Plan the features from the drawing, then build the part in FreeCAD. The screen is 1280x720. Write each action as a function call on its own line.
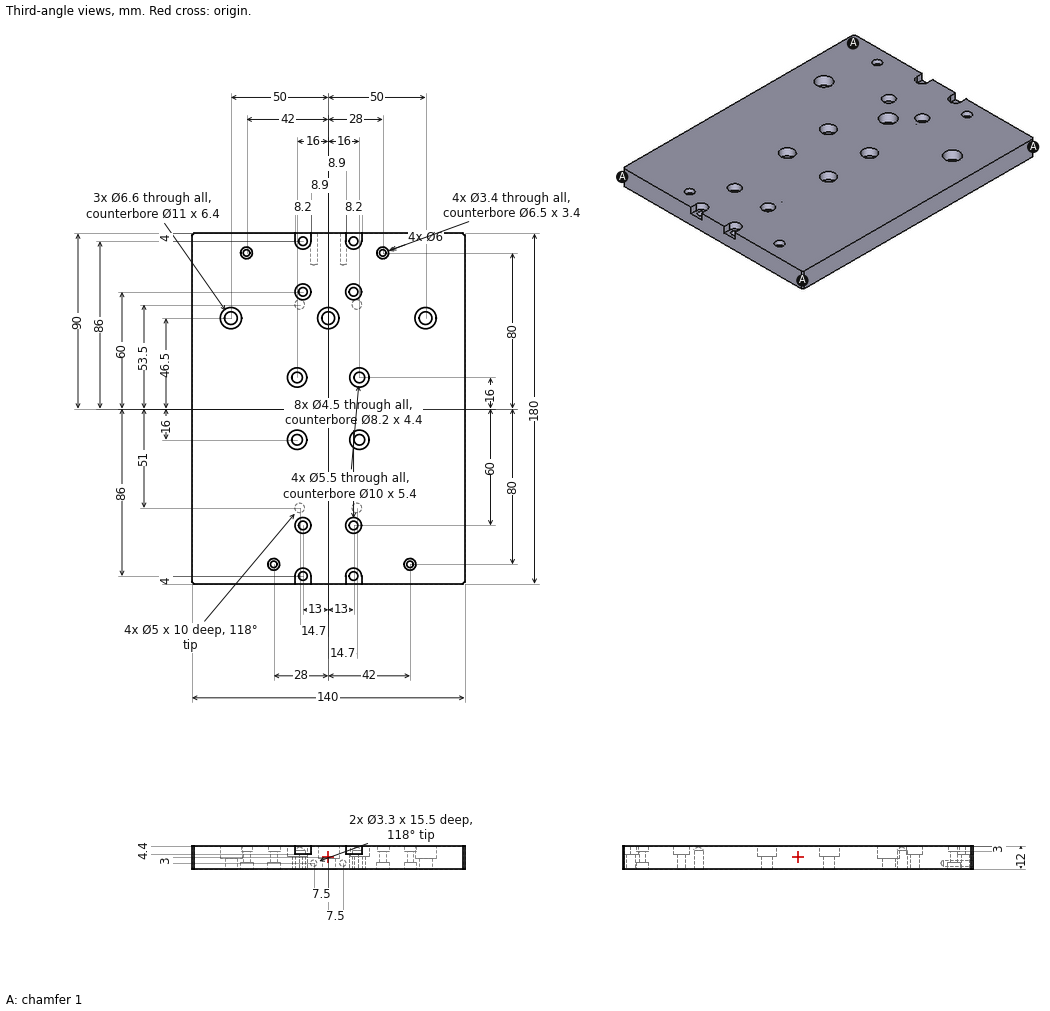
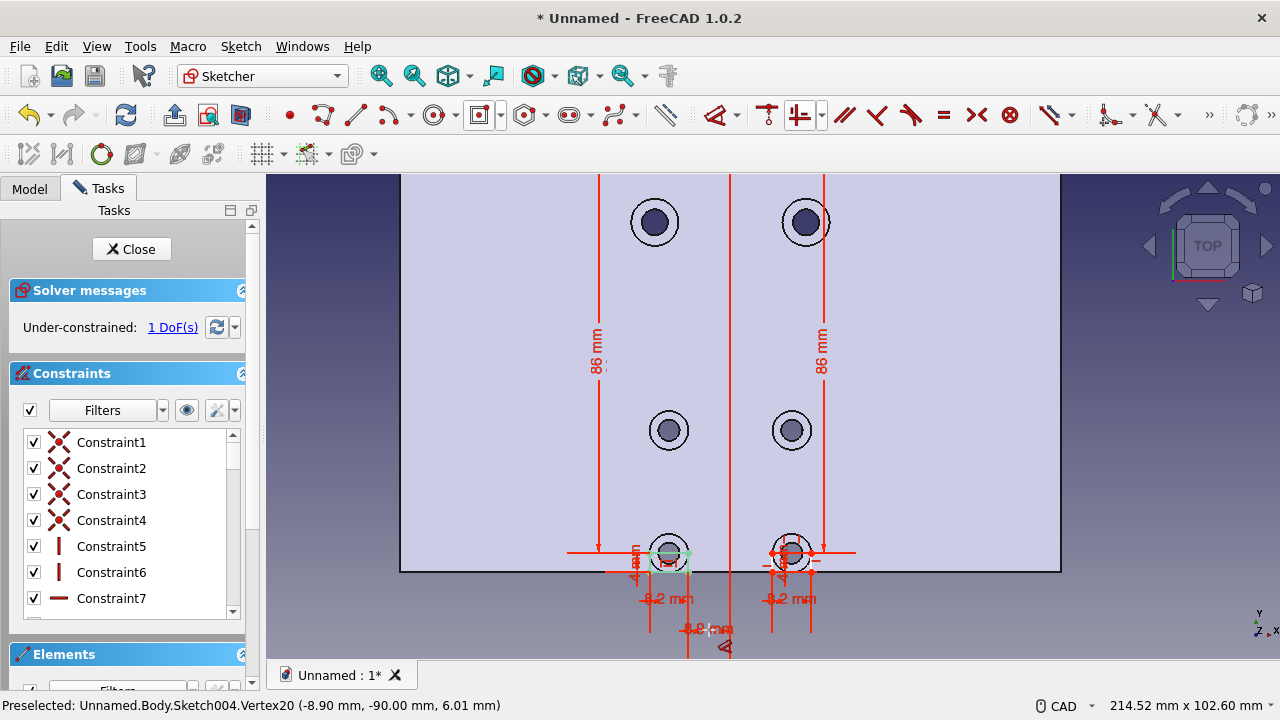
click(772, 553)
click(751, 587)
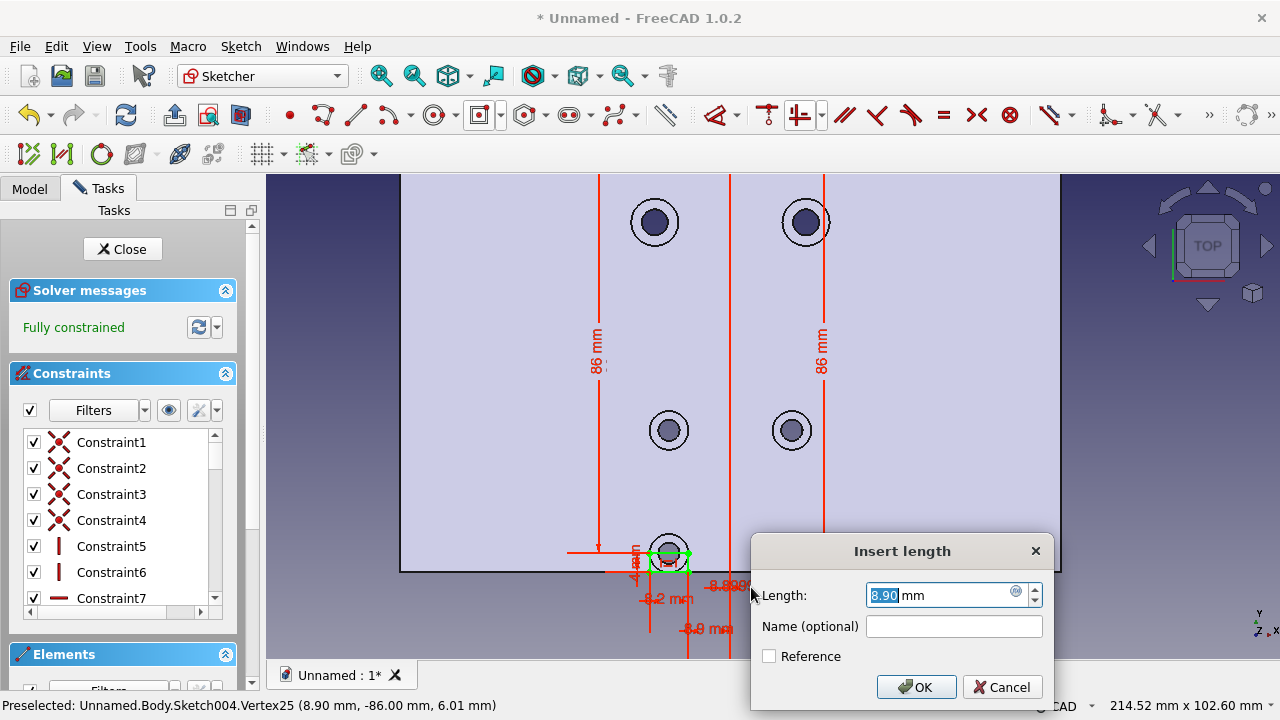
text(8.9)
key(Return)
key(Escape)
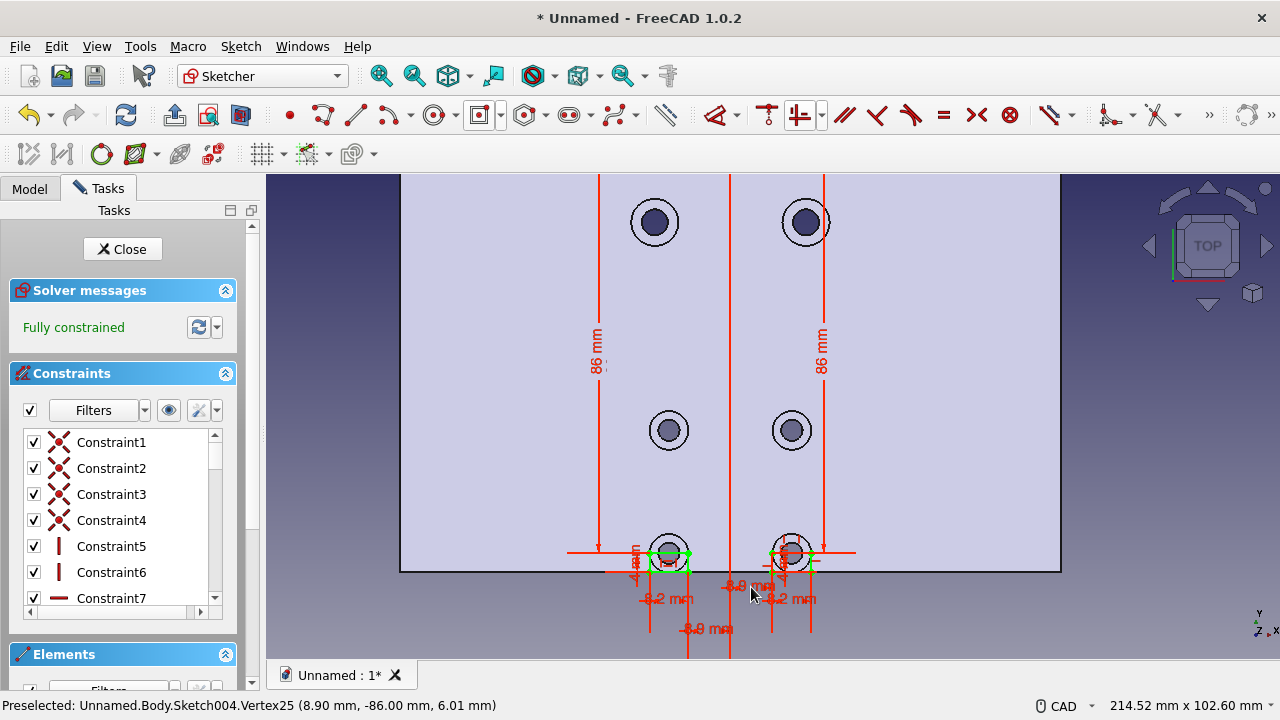
click(123, 249)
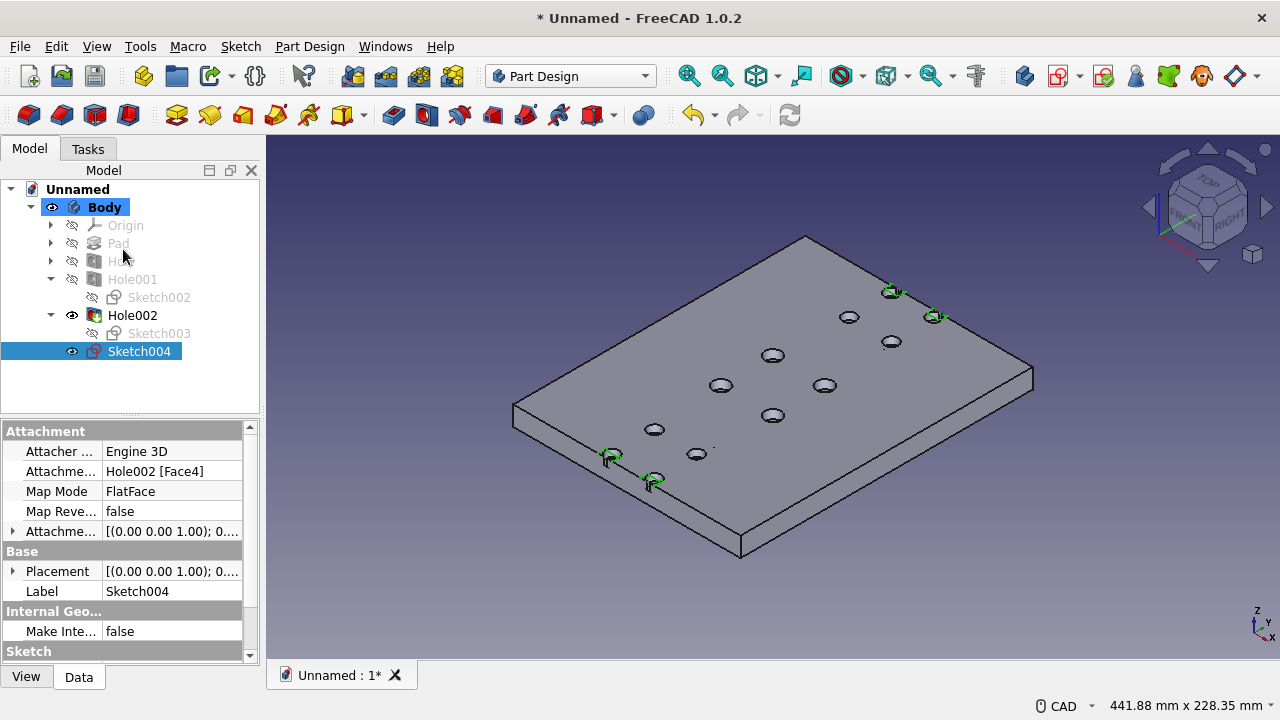
click(394, 116)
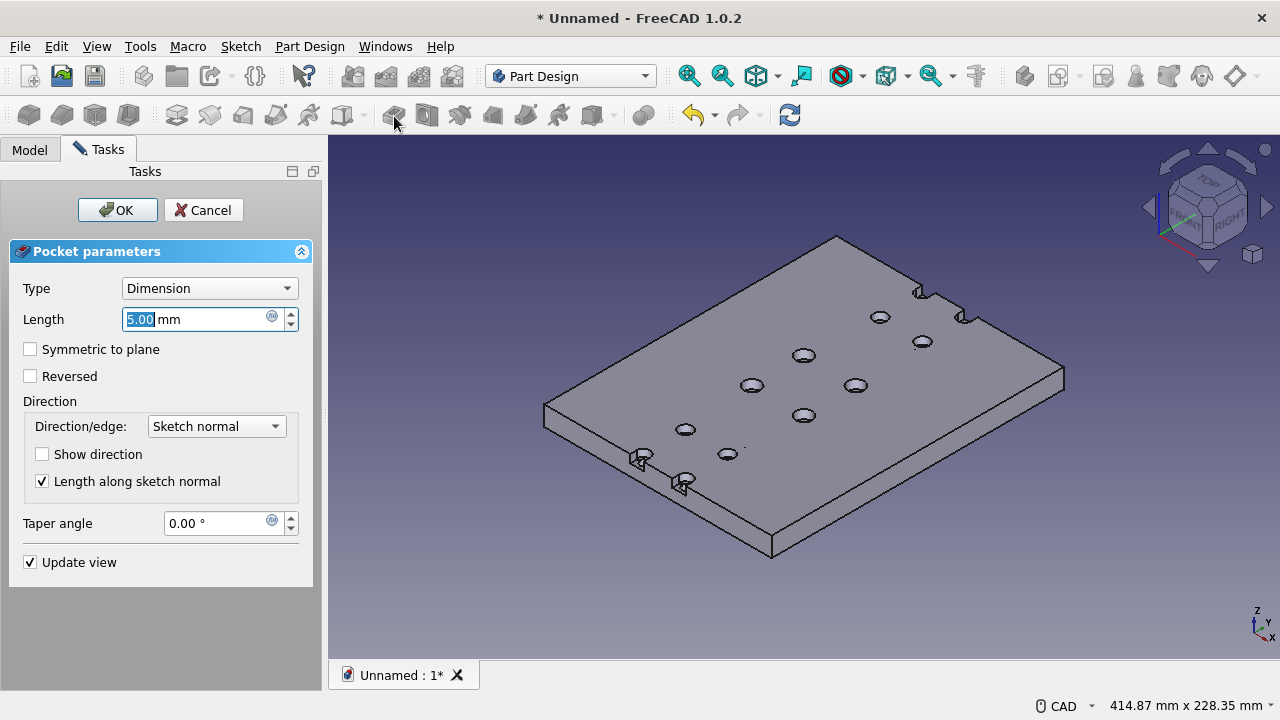
text(4.4)
key(Tab)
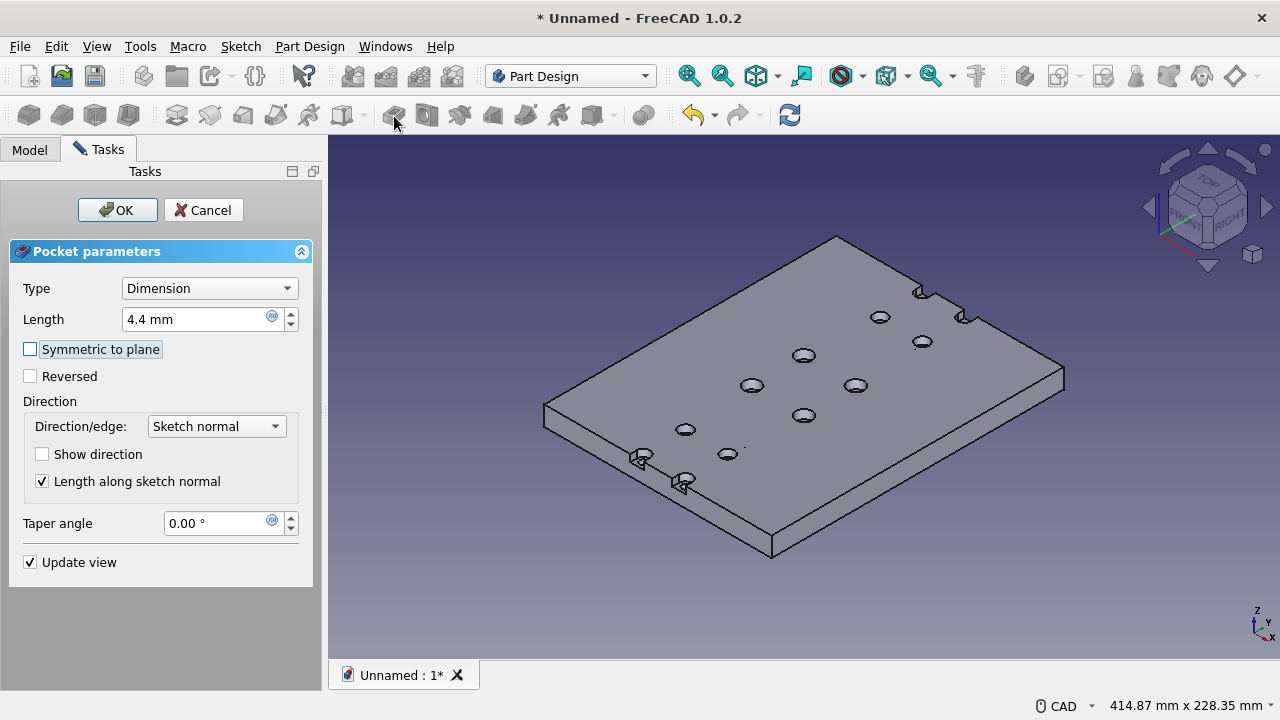
click(118, 210)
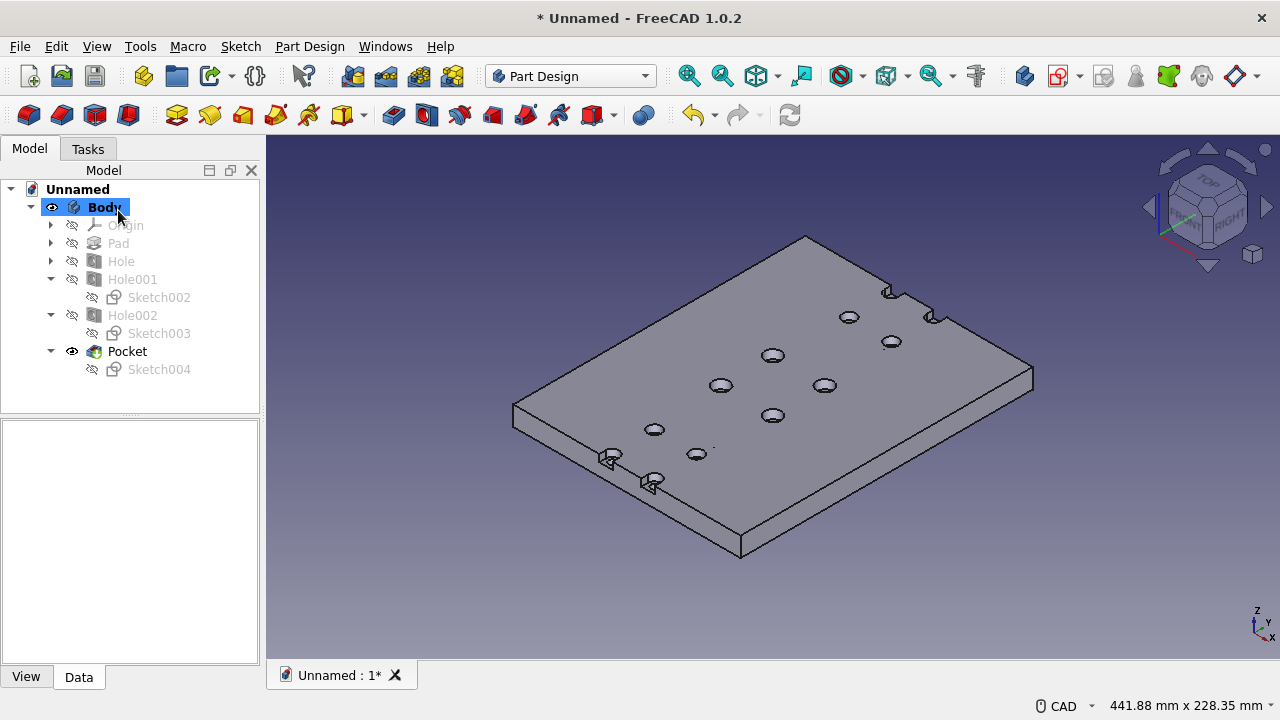
key(4)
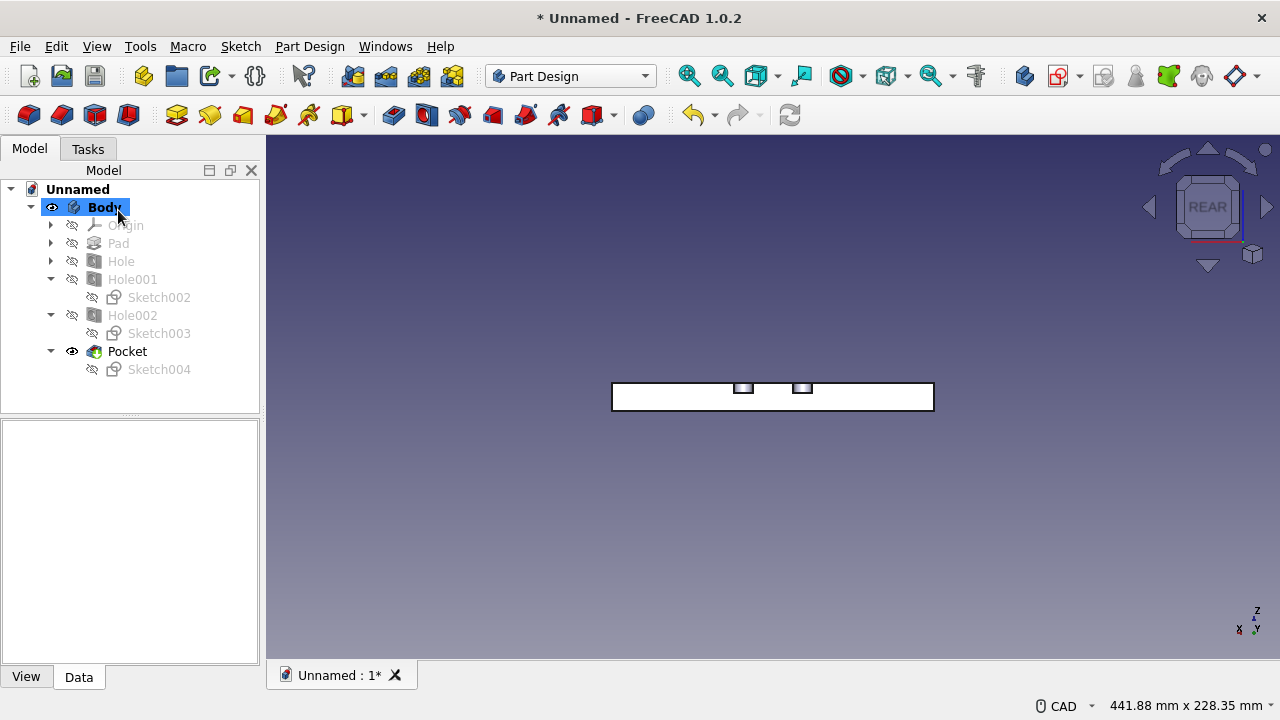
click(690, 76)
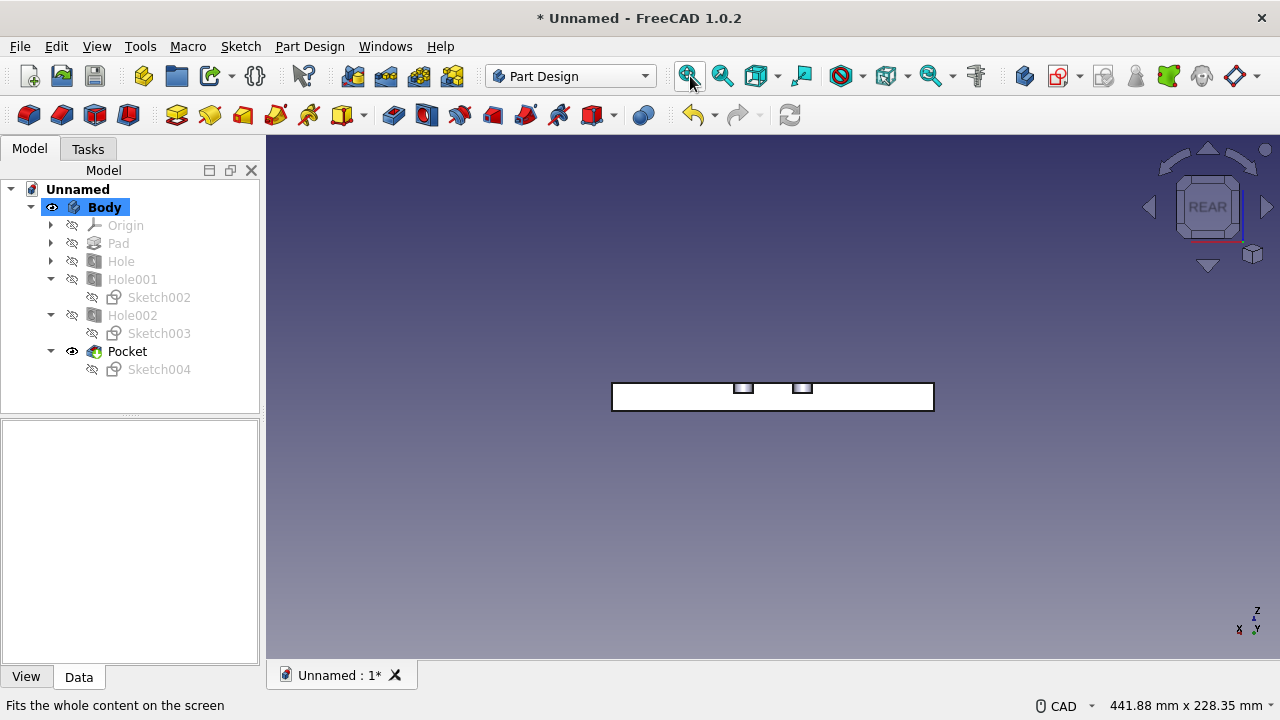
click(635, 396)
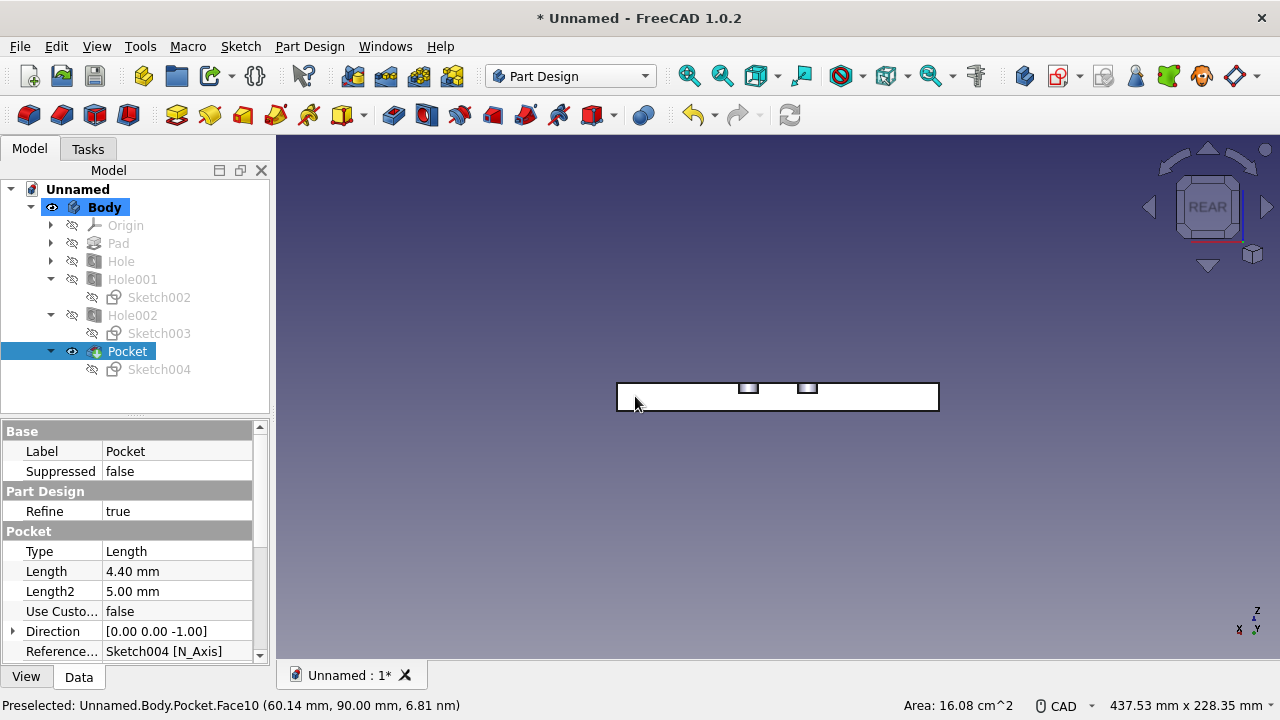
click(1058, 76)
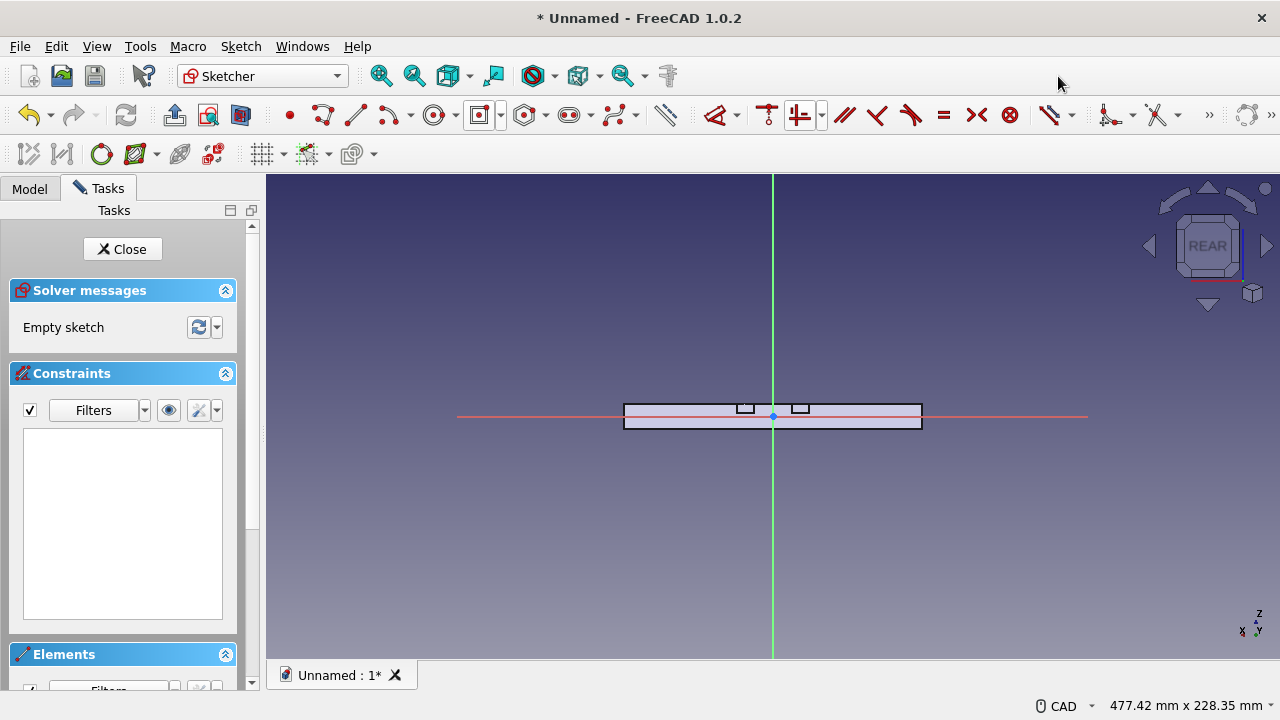
scroll(777, 422, up, 14)